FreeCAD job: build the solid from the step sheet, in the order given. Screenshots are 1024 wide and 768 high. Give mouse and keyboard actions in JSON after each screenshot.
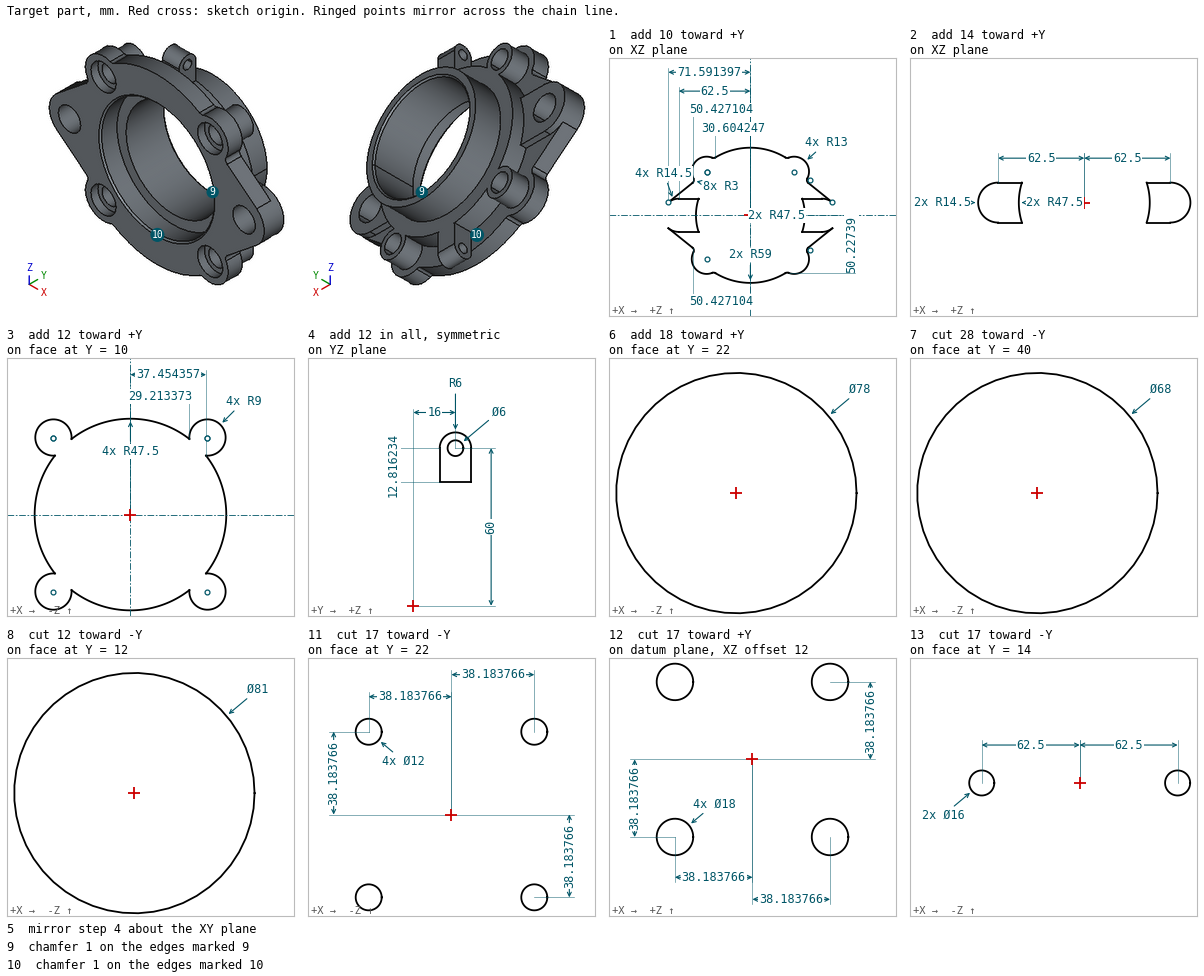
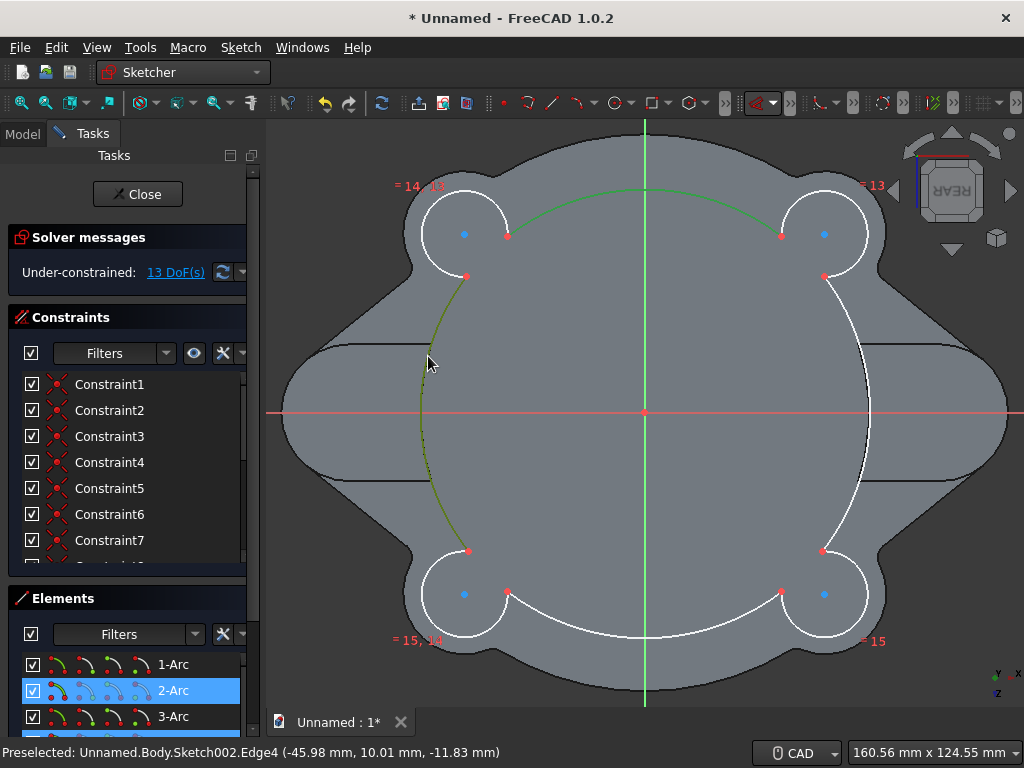
{"action": "left_click", "coordinate": [586, 631]}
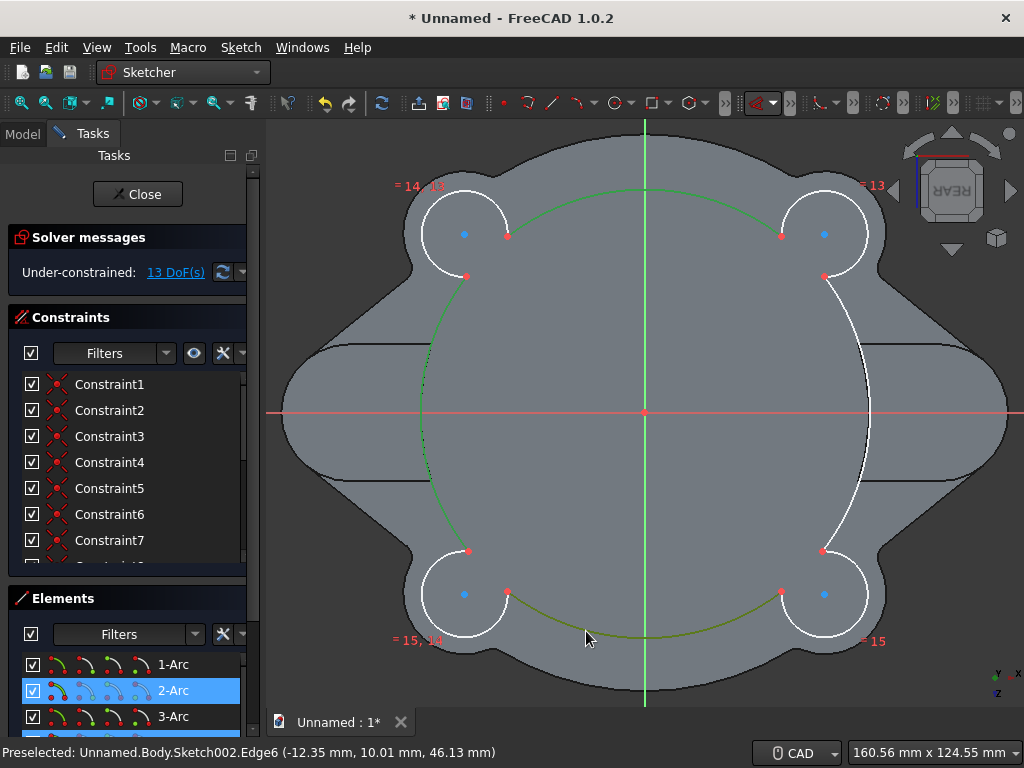
{"action": "left_click", "coordinate": [852, 501]}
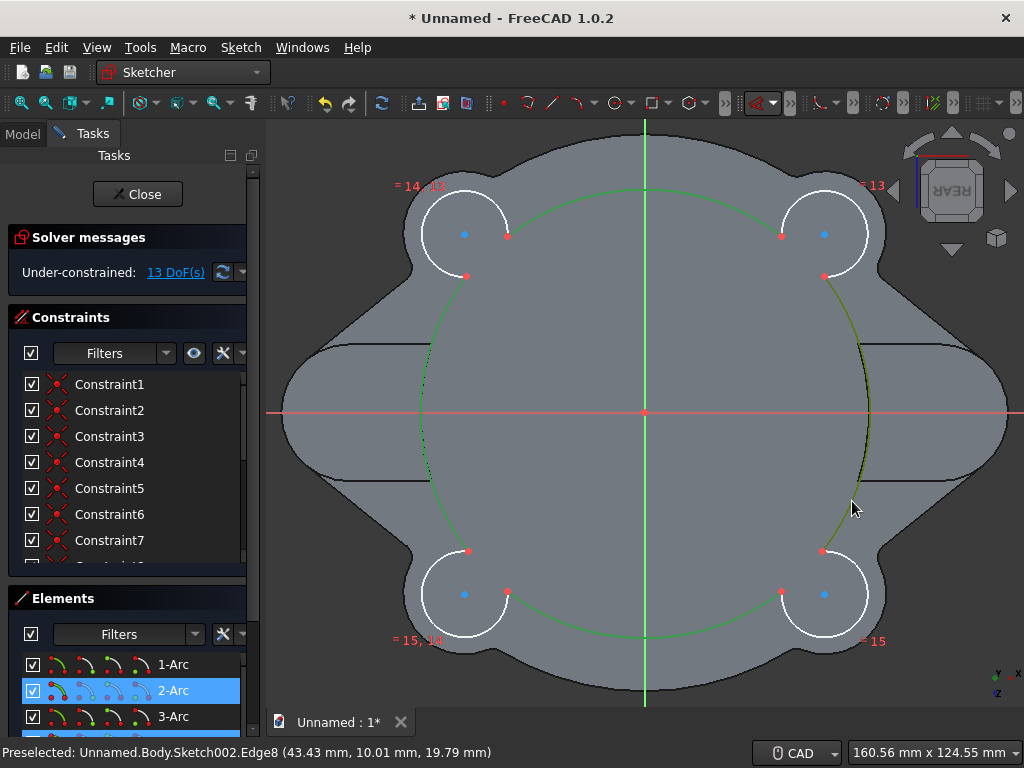
{"action": "key", "text": "e"}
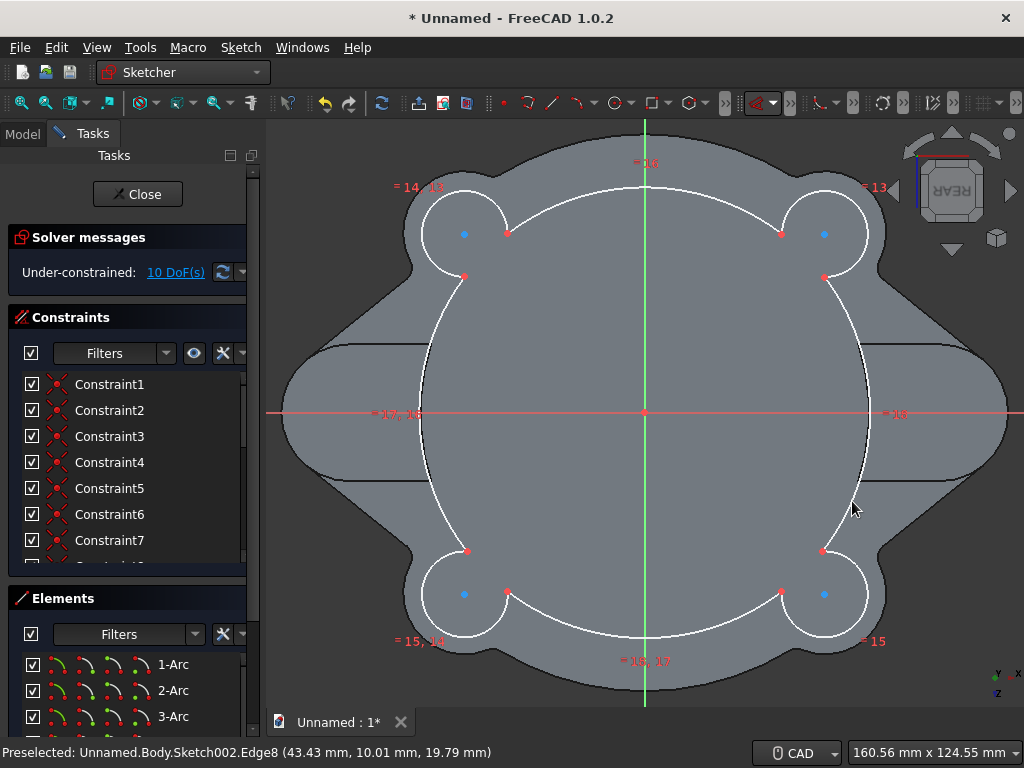
{"action": "left_click", "coordinate": [825, 234]}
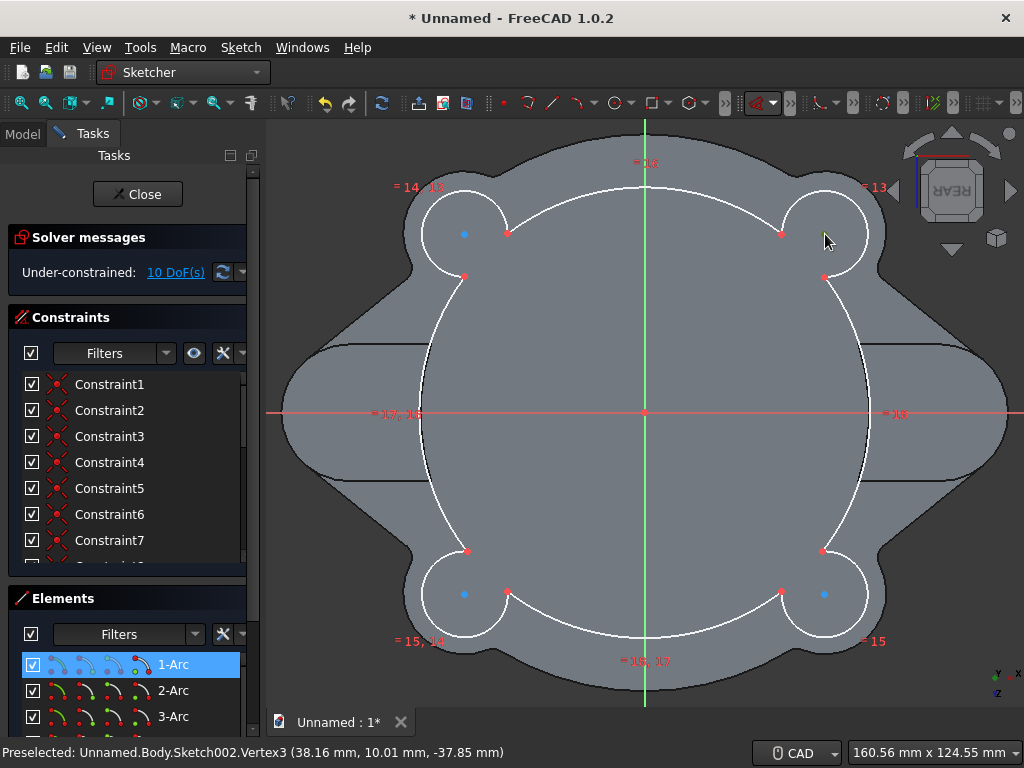
{"action": "left_click", "coordinate": [465, 234]}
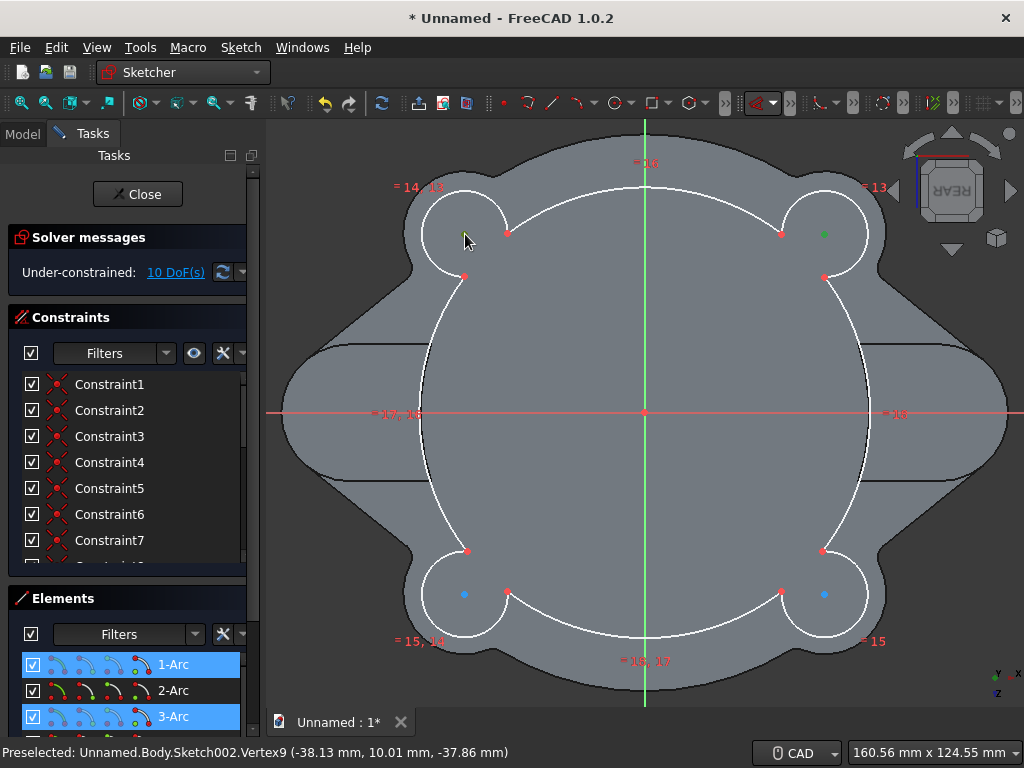
{"action": "left_click", "coordinate": [645, 603]}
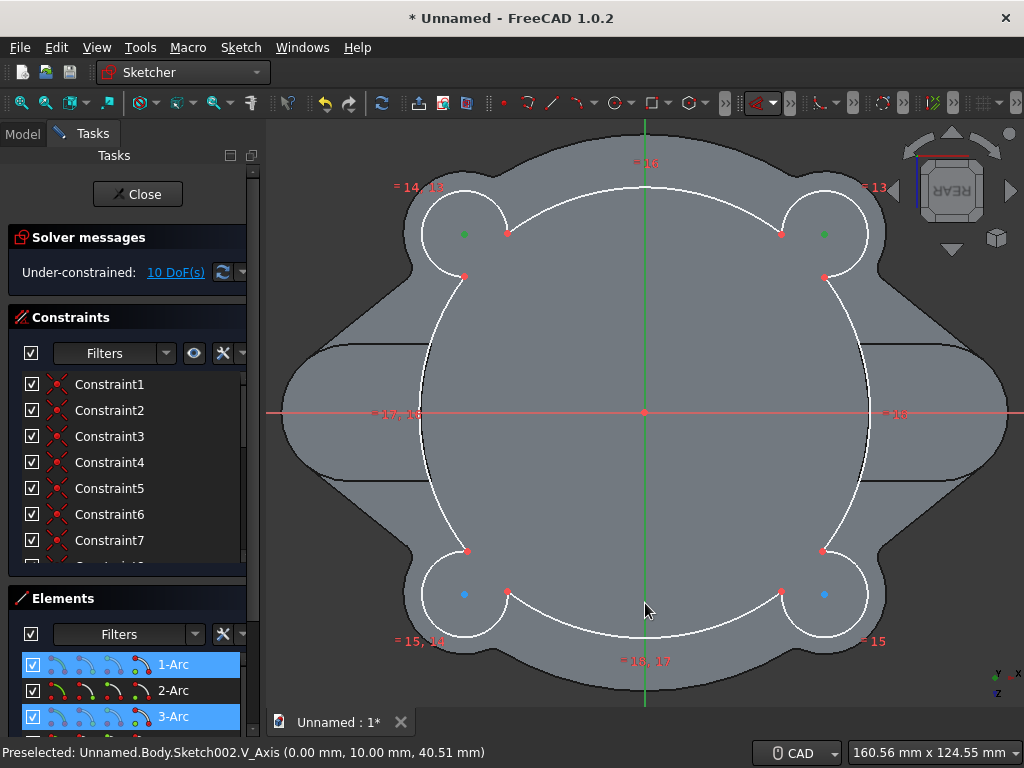
{"action": "key", "text": "s"}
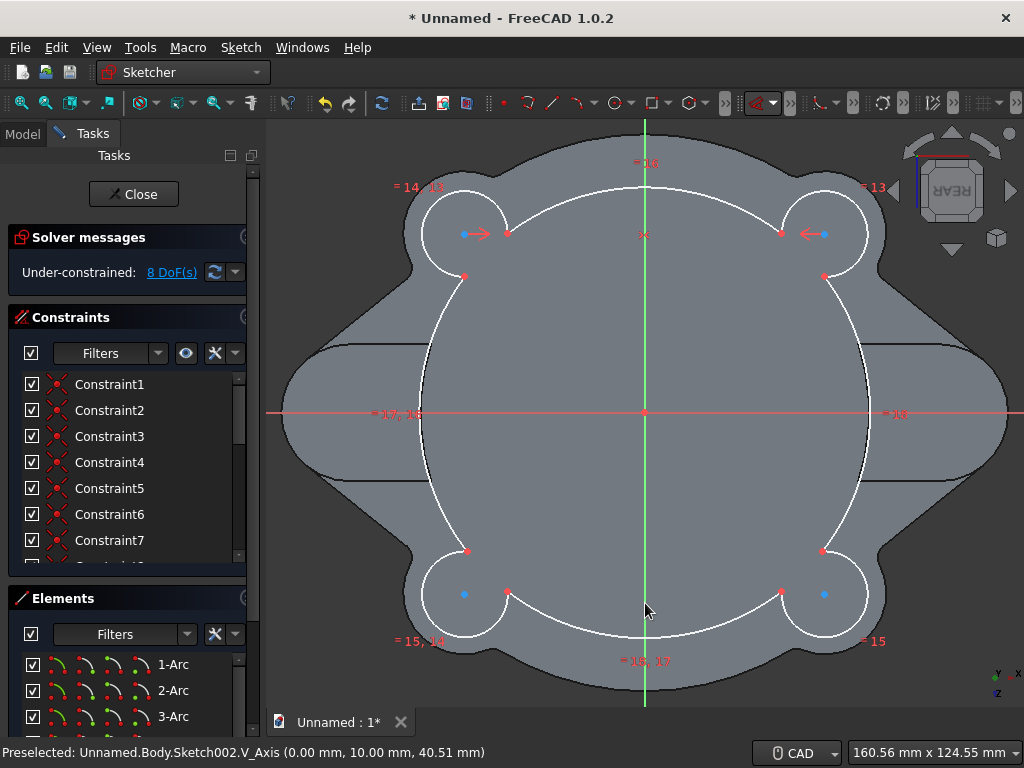
{"action": "left_click", "coordinate": [465, 234]}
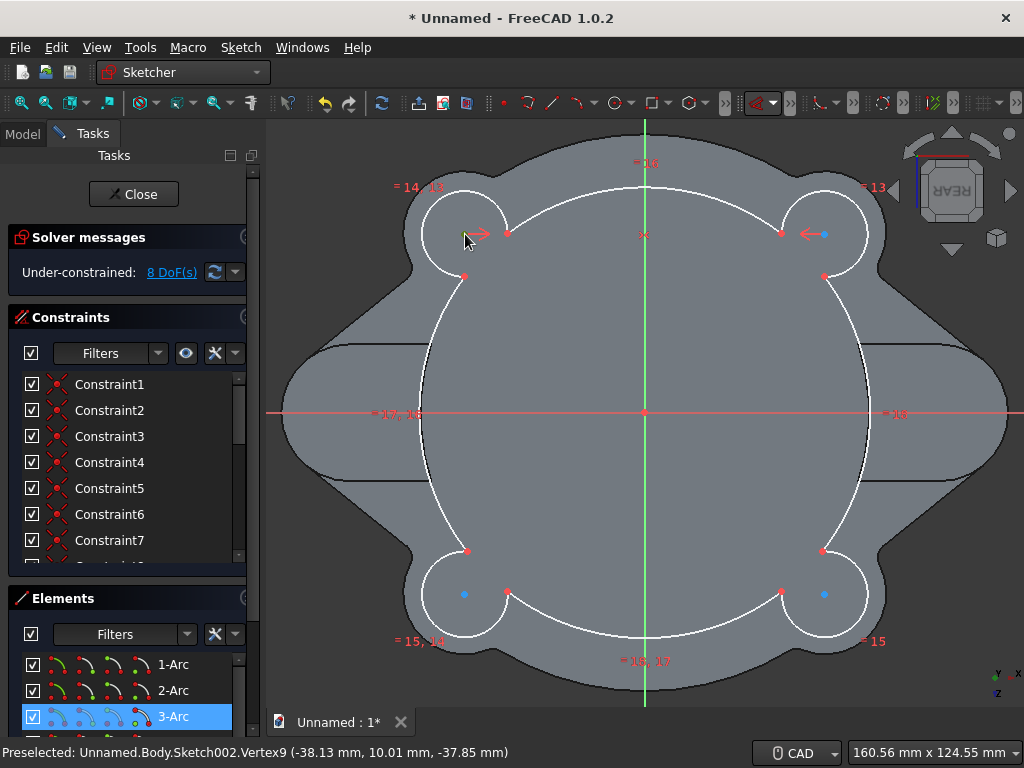
{"action": "left_click", "coordinate": [465, 594]}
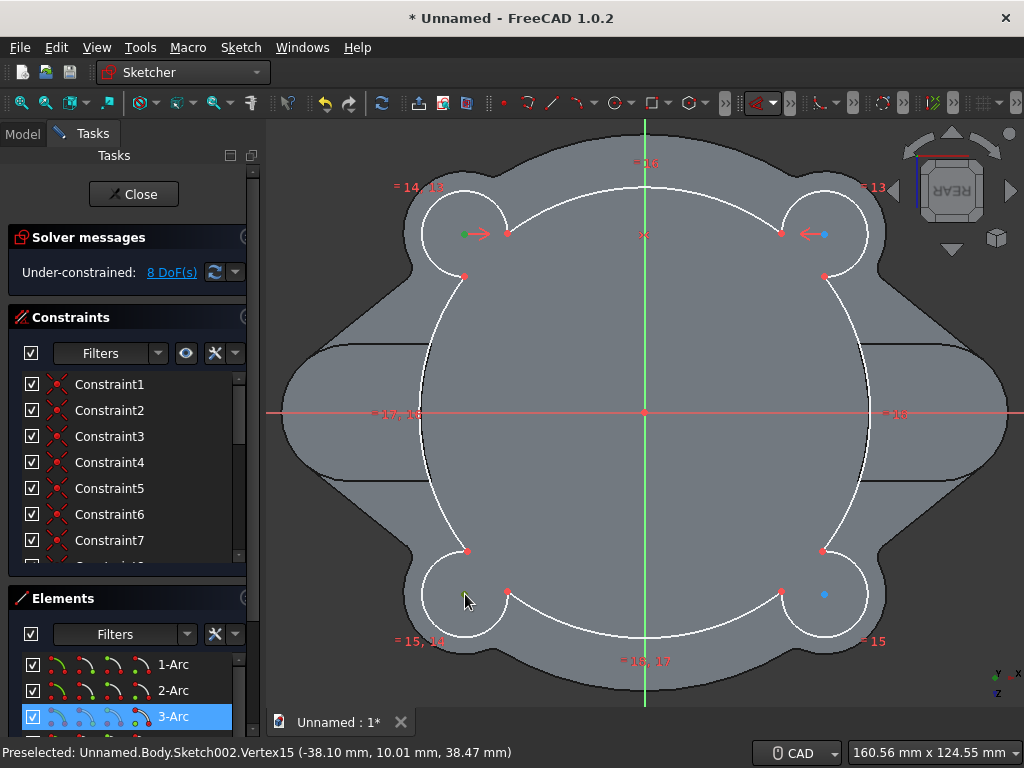
{"action": "left_click", "coordinate": [334, 413]}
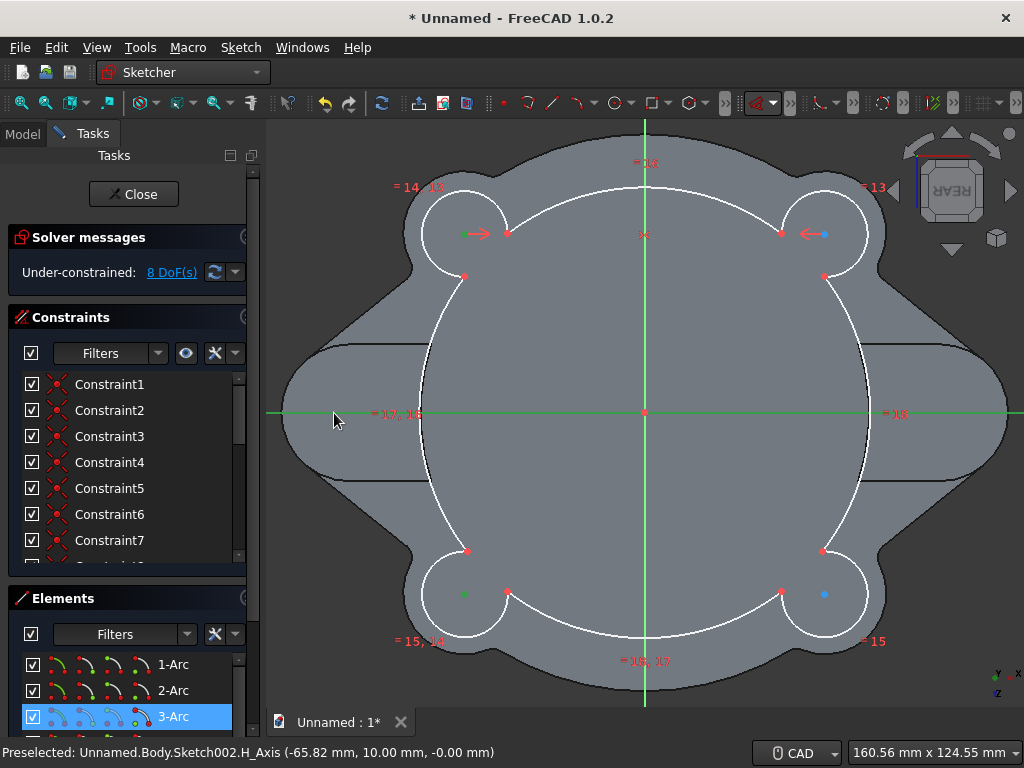
{"action": "key", "text": "s"}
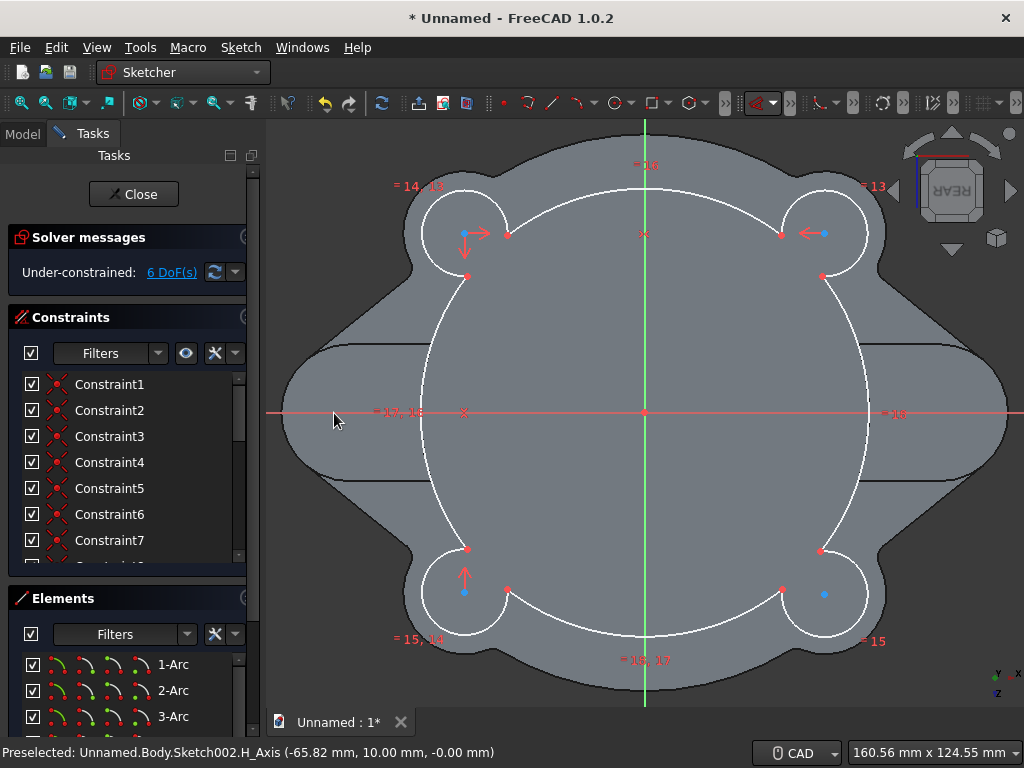
{"action": "left_click", "coordinate": [825, 233]}